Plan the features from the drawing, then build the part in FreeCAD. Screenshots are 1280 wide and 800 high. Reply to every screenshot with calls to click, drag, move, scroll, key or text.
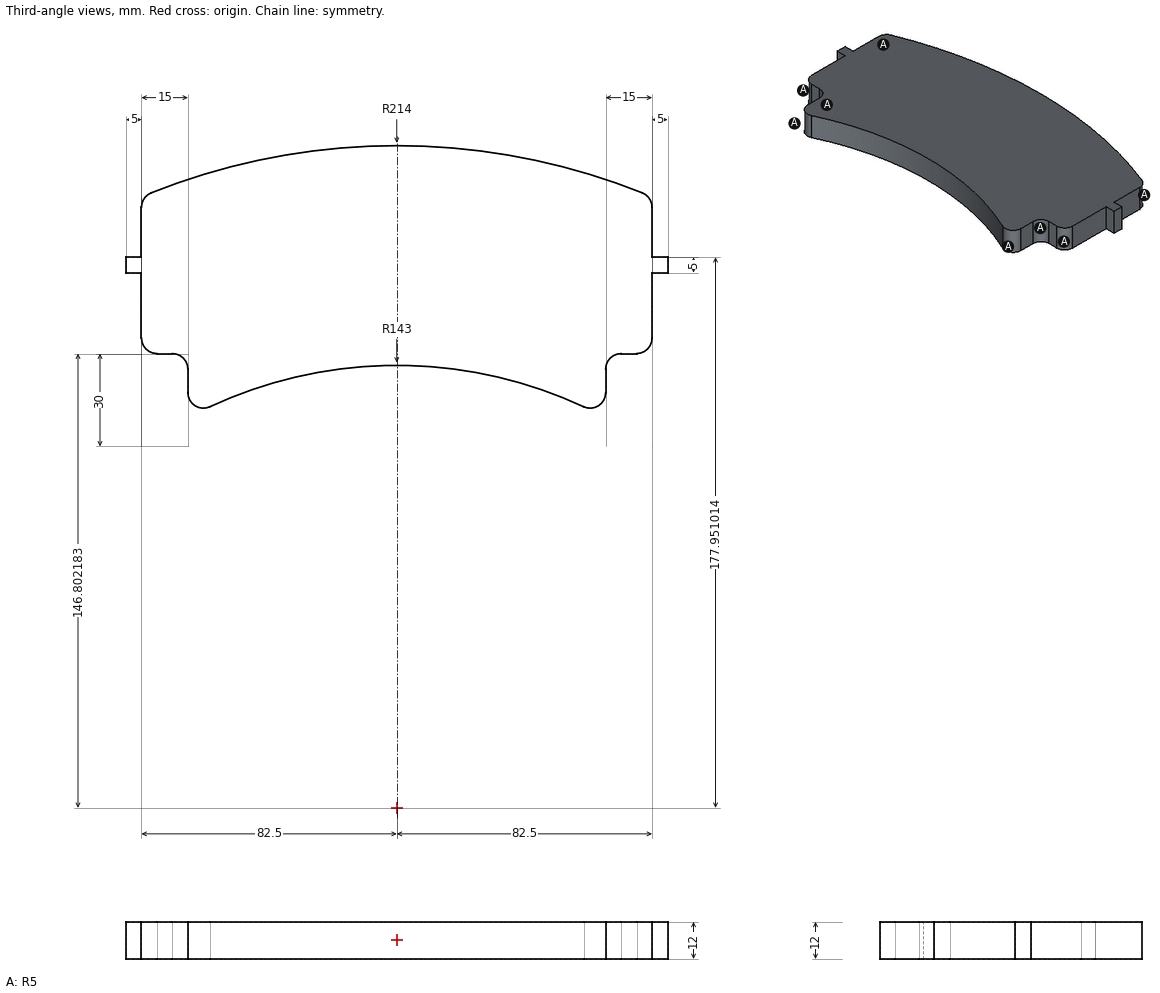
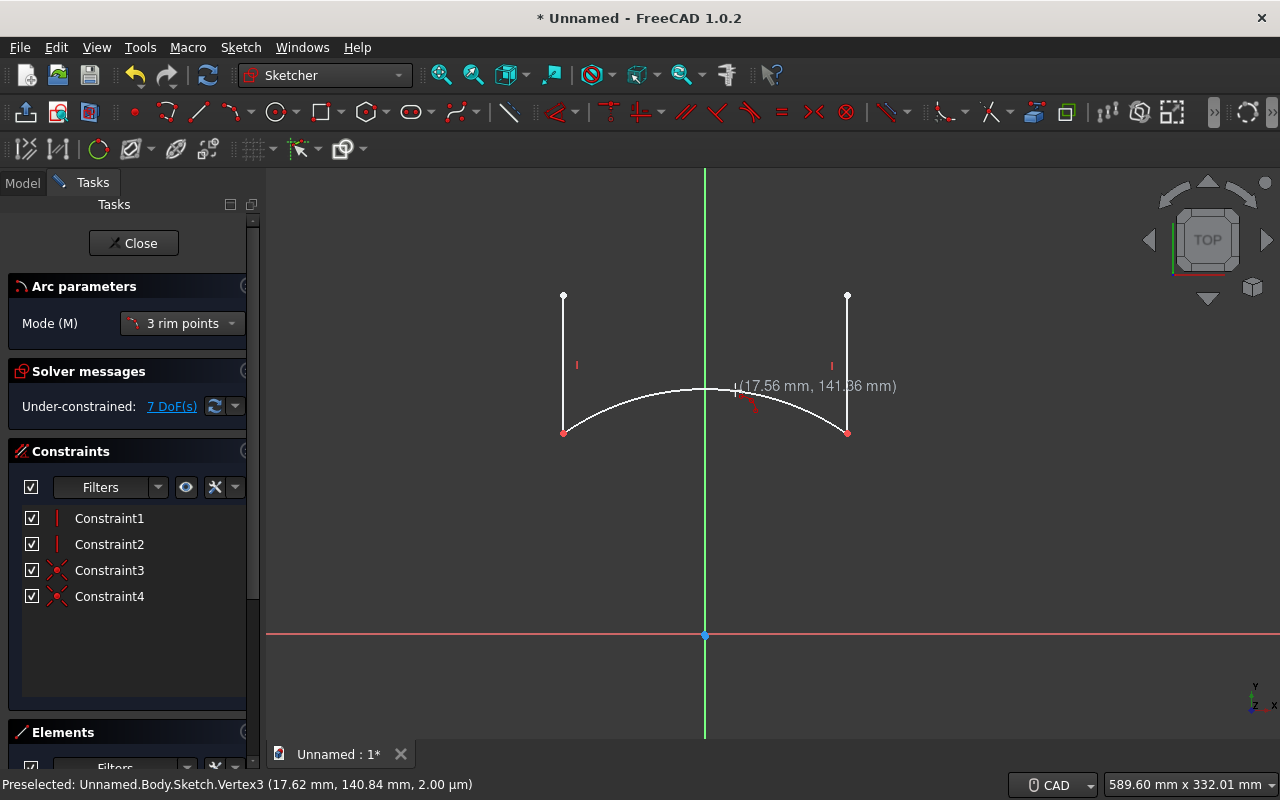
click(847, 296)
click(563, 296)
click(734, 267)
key(Escape)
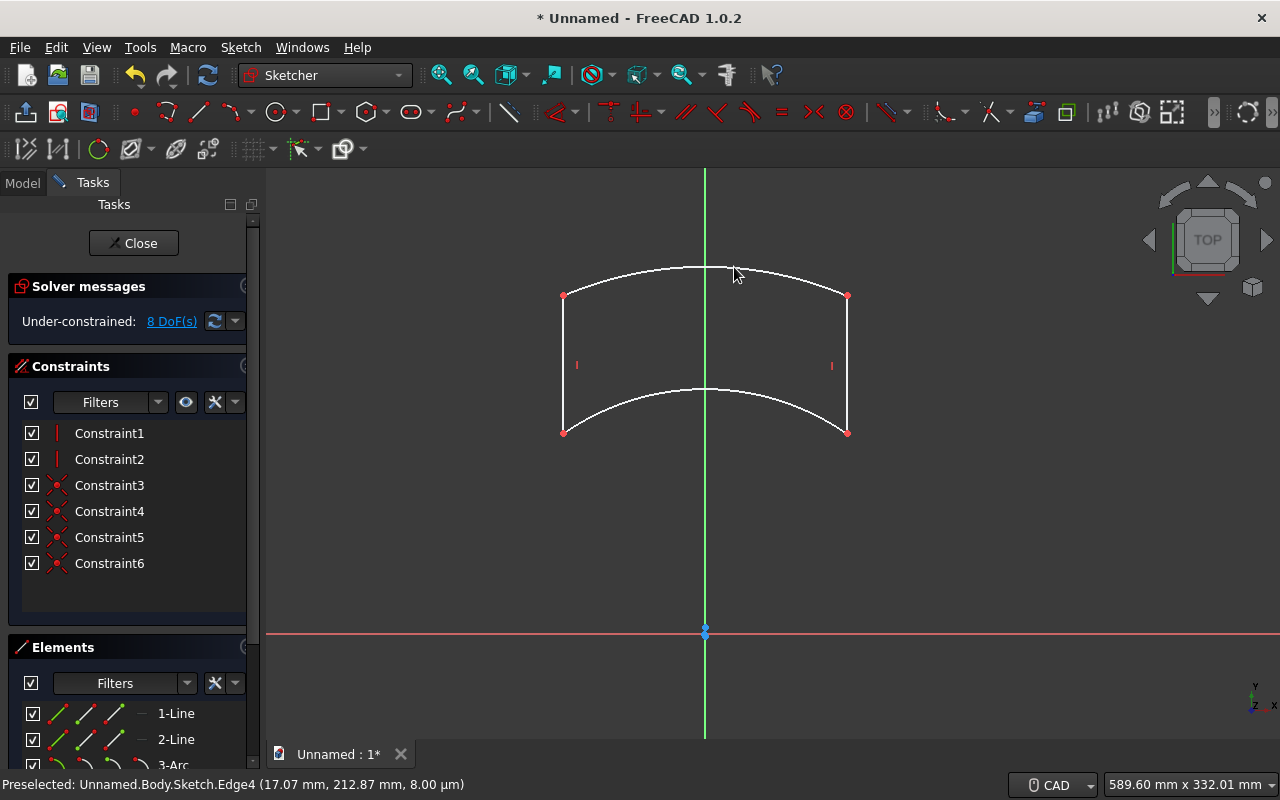
click(765, 397)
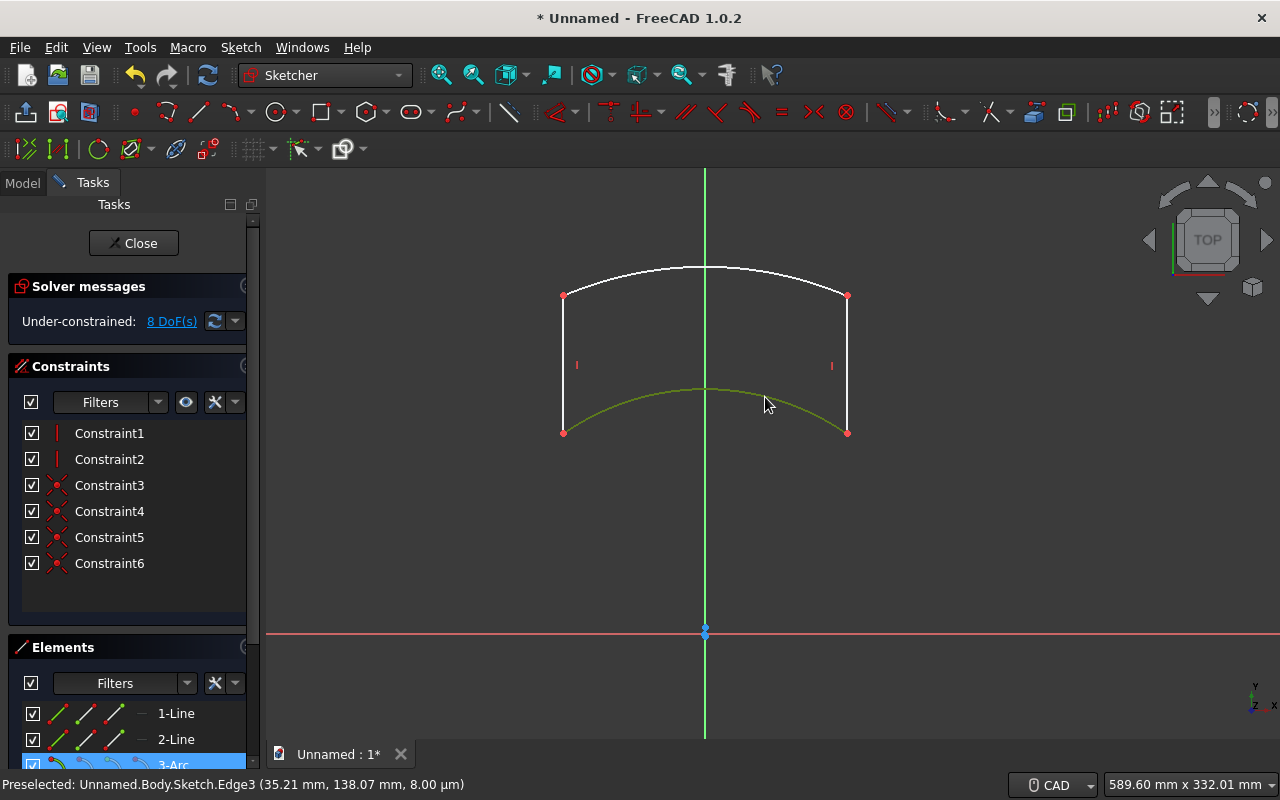
click(763, 272)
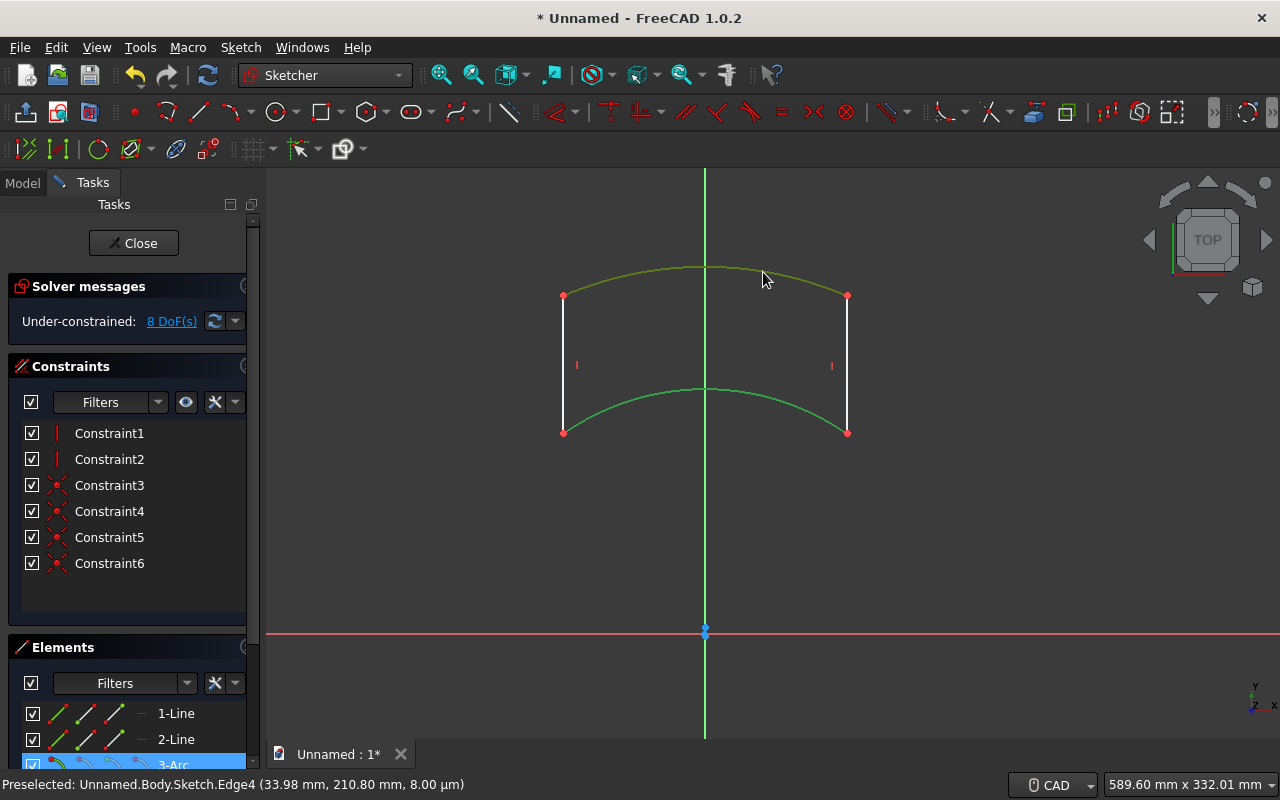
click(610, 112)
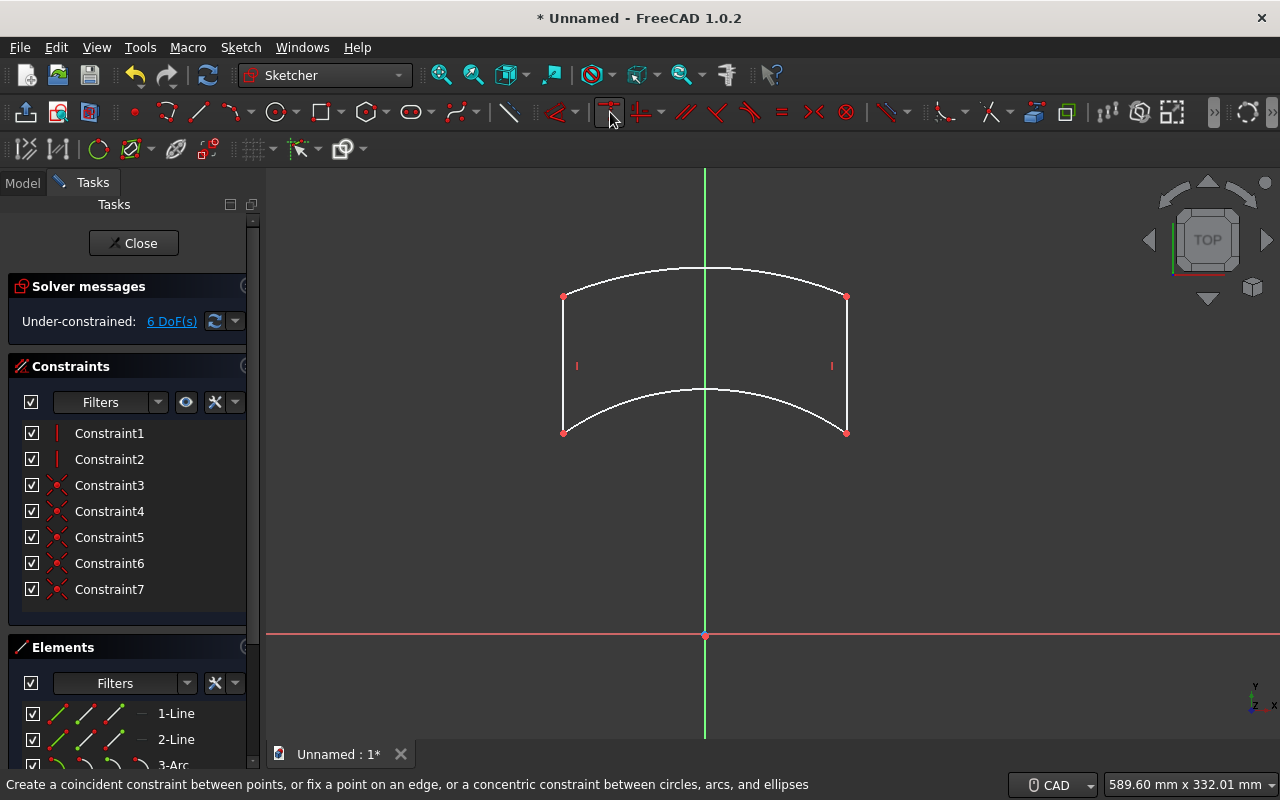
drag(695, 624, 715, 646)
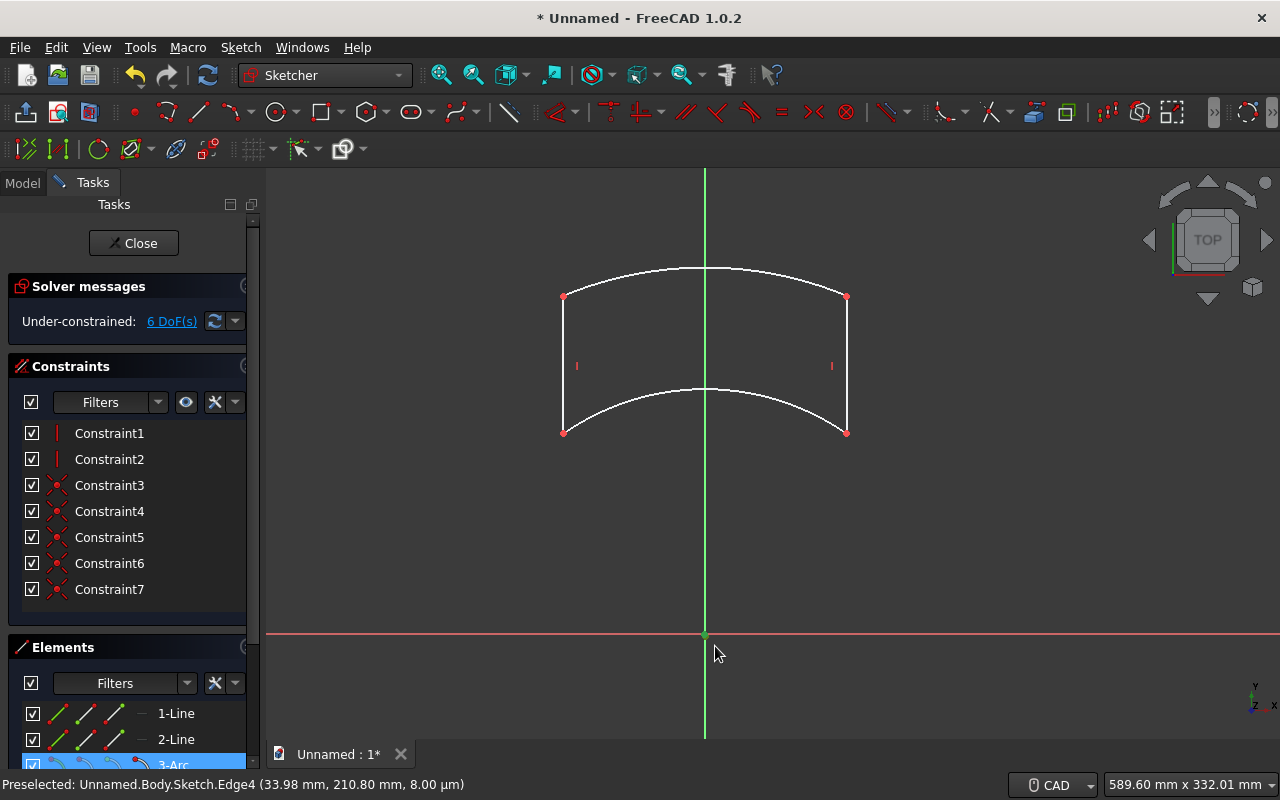
click(610, 112)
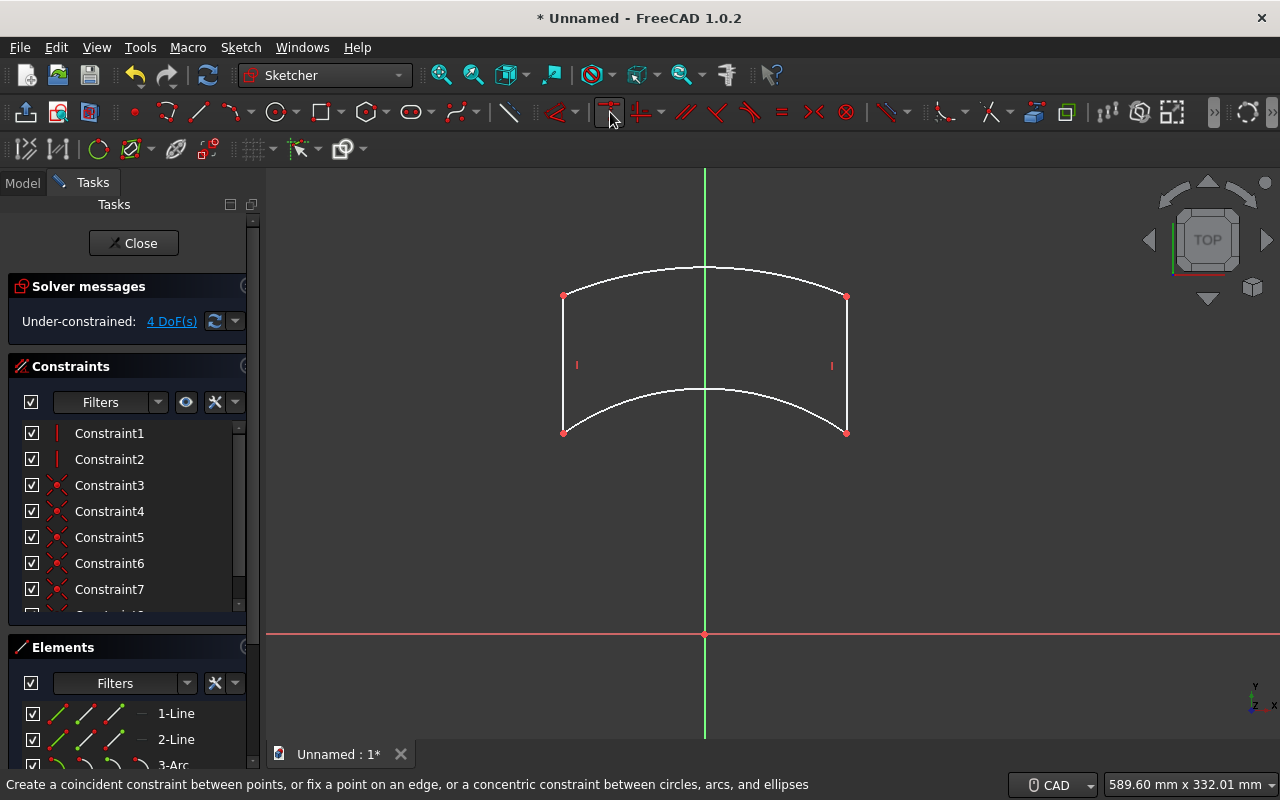
click(556, 112)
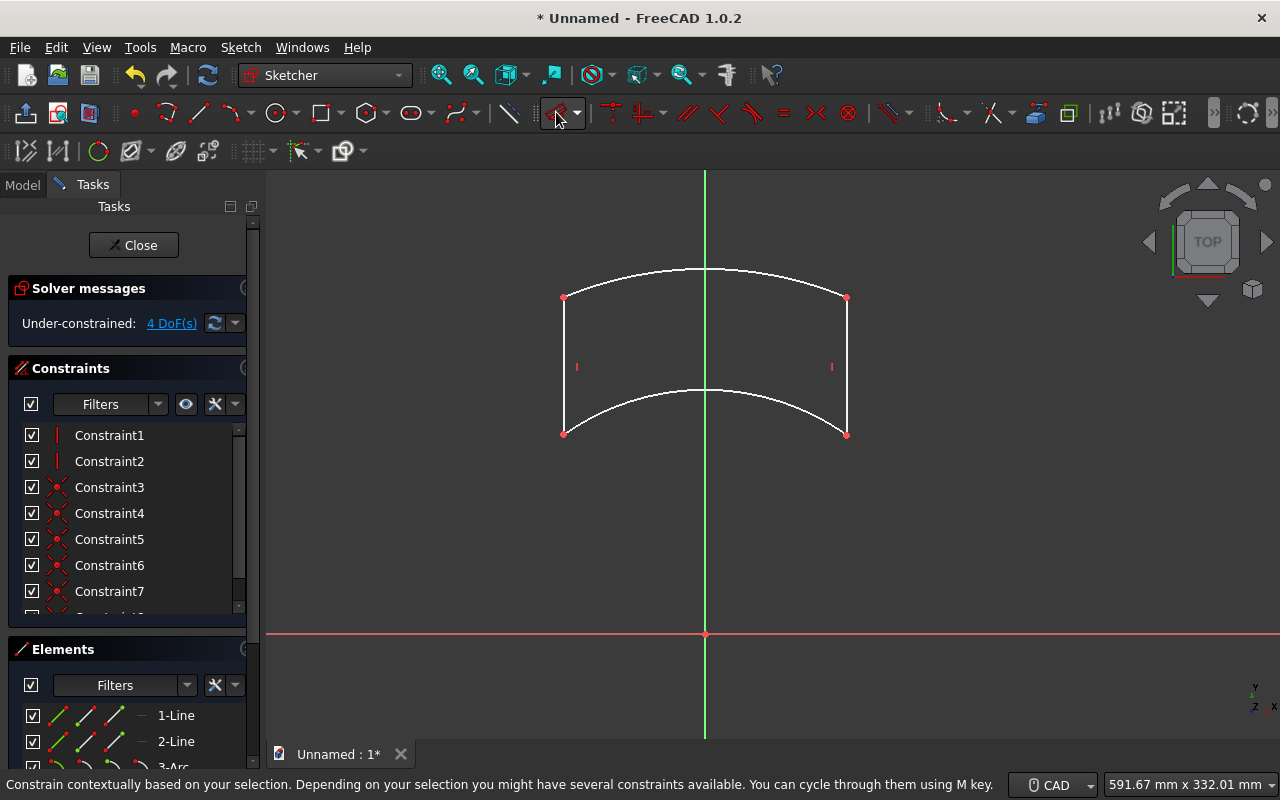
click(765, 397)
click(773, 366)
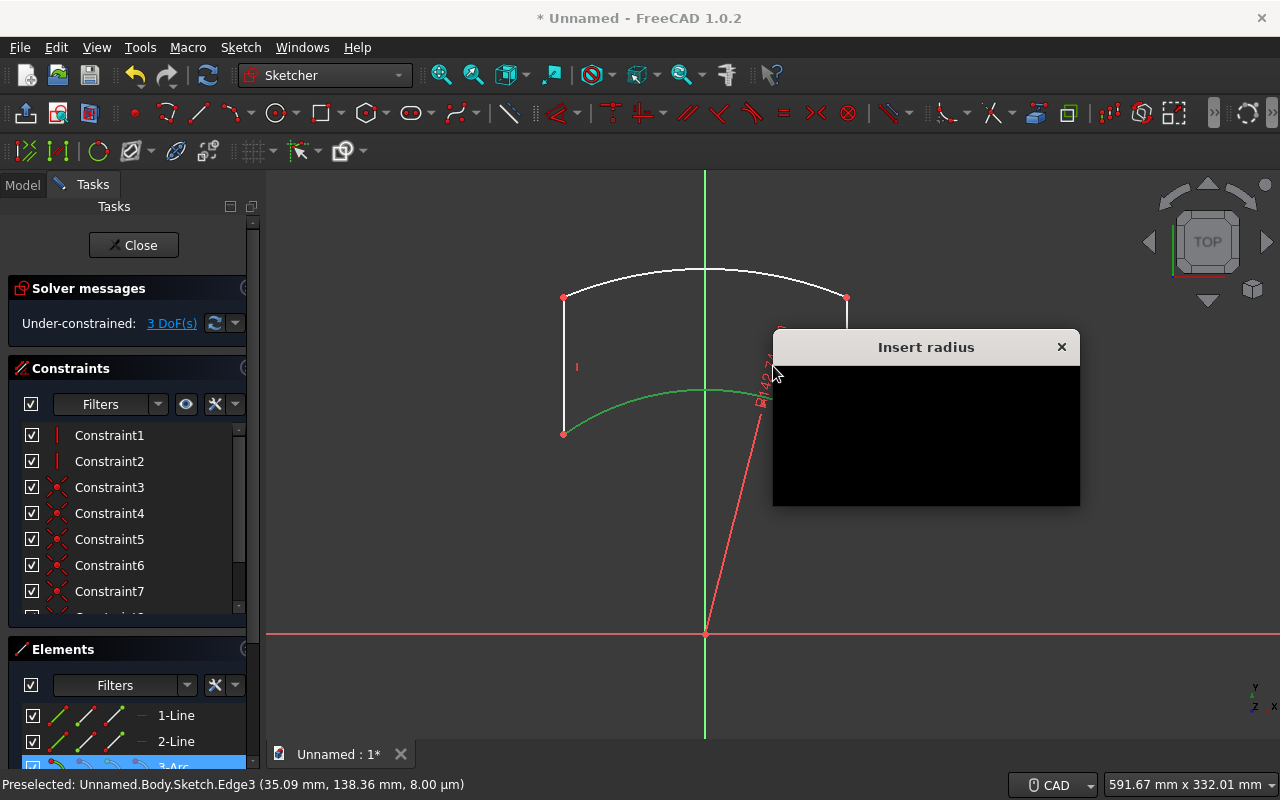
text(143)
key(Return)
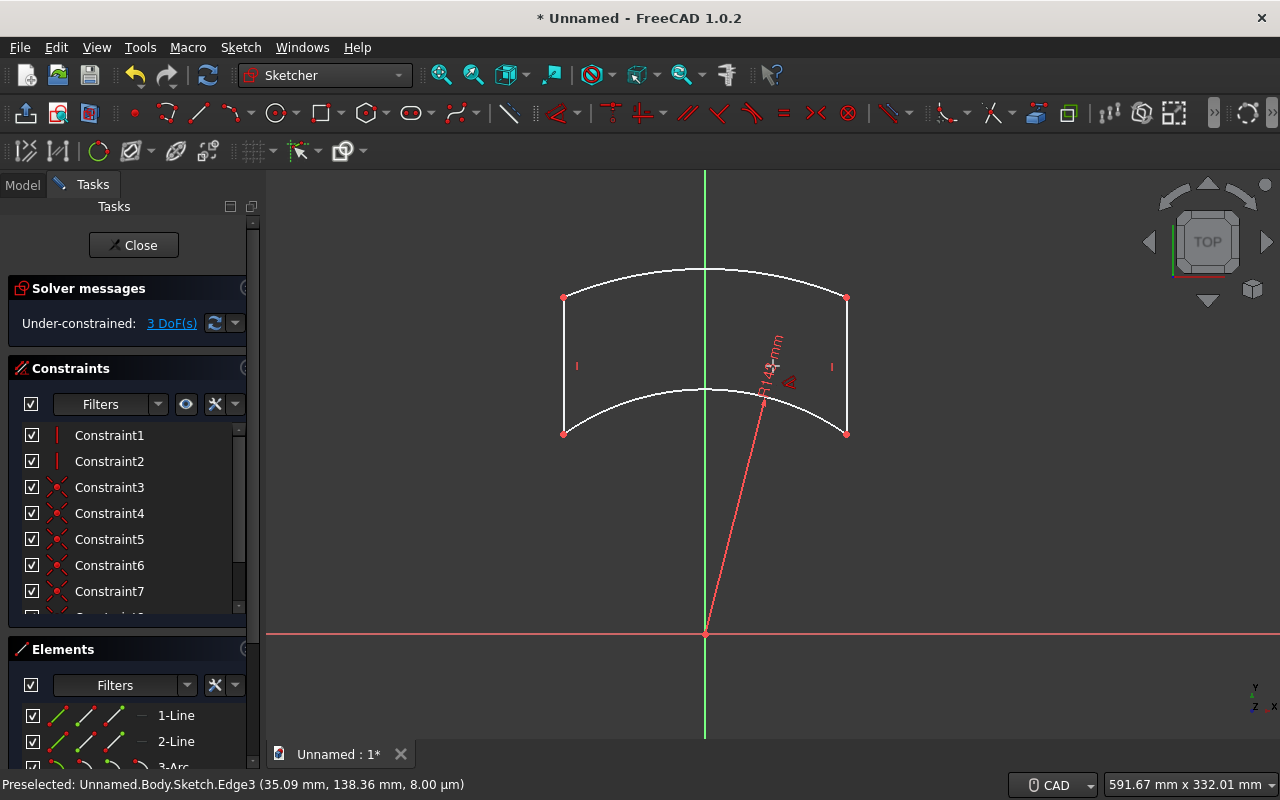
click(763, 274)
click(768, 242)